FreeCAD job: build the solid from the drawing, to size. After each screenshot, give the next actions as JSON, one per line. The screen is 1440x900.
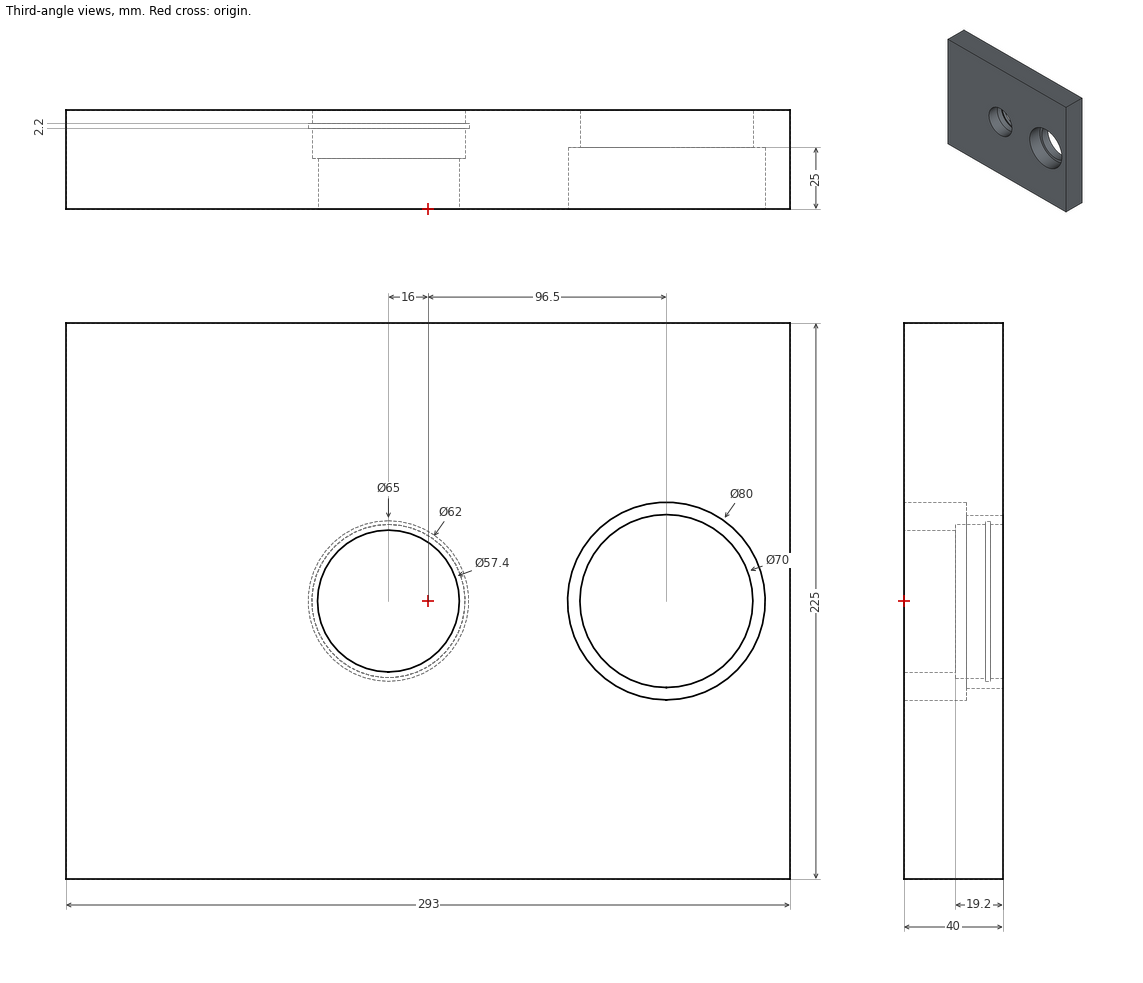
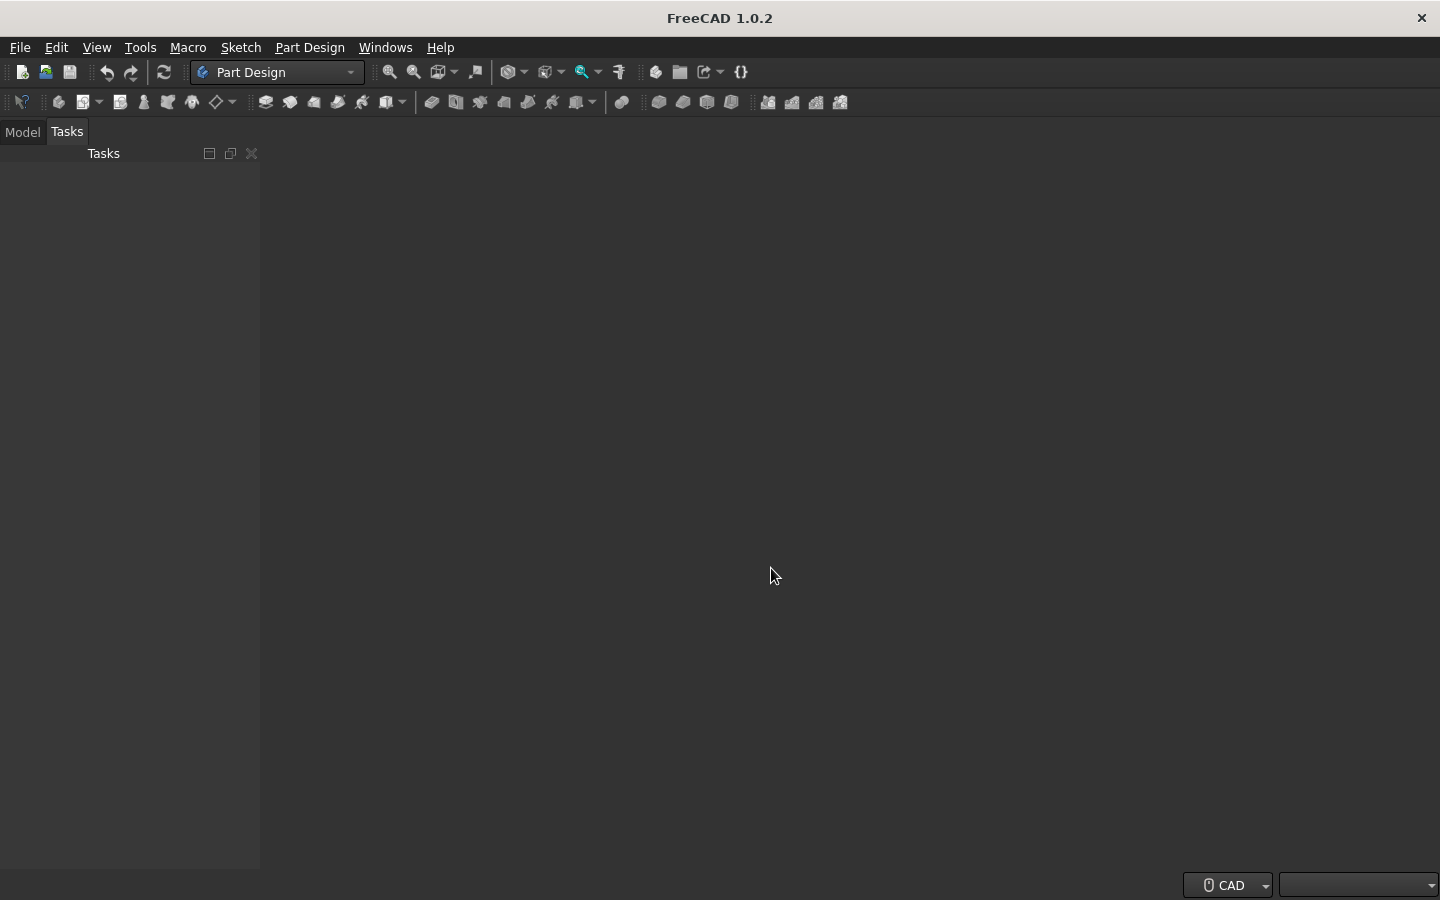
{"action": "left_click", "coordinate": [22, 72]}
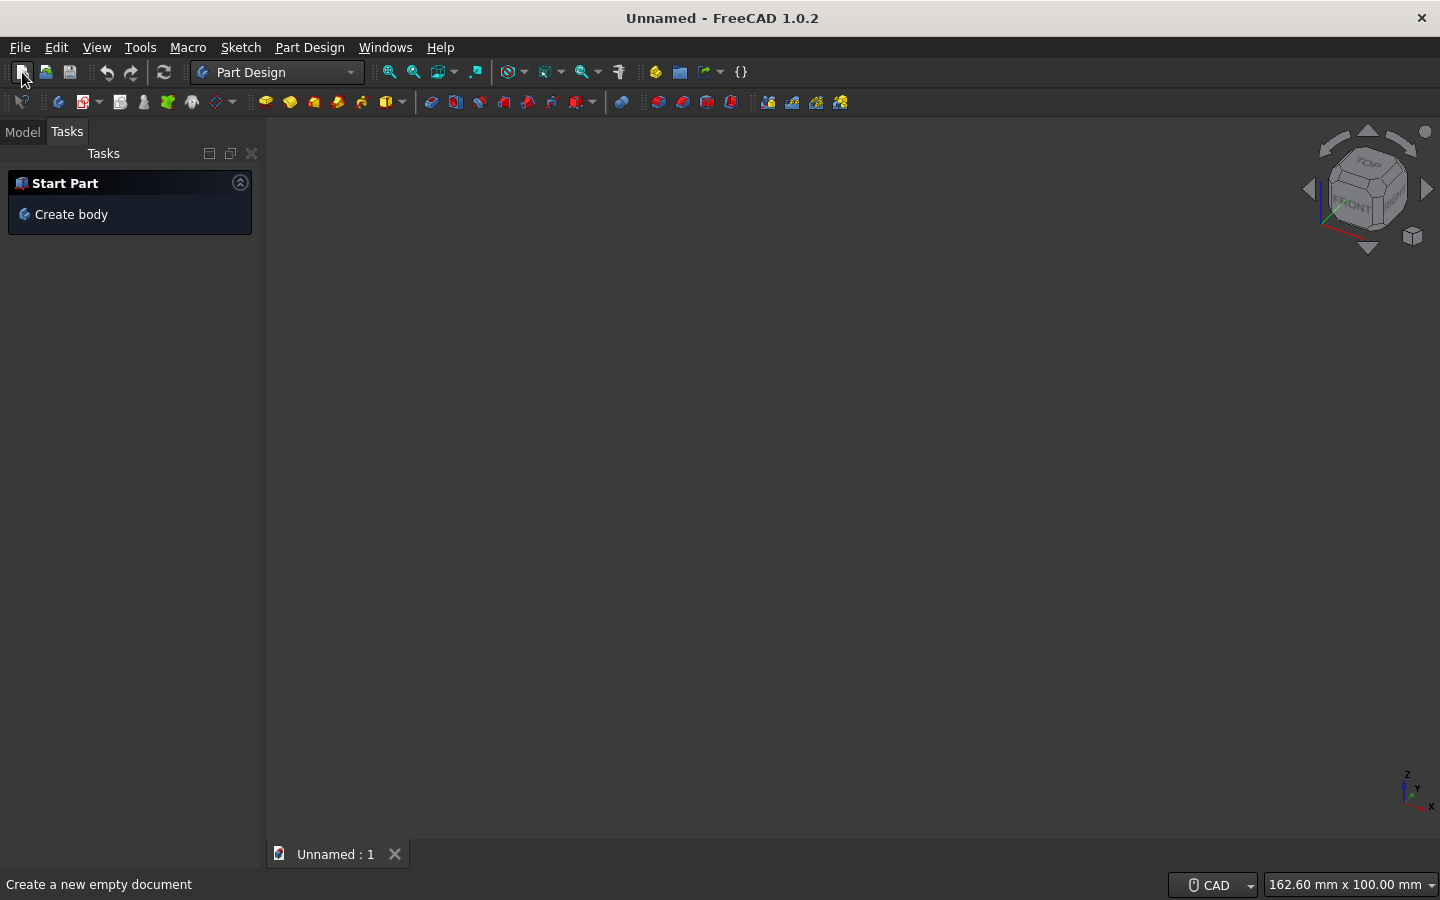
{"action": "left_click", "coordinate": [84, 102]}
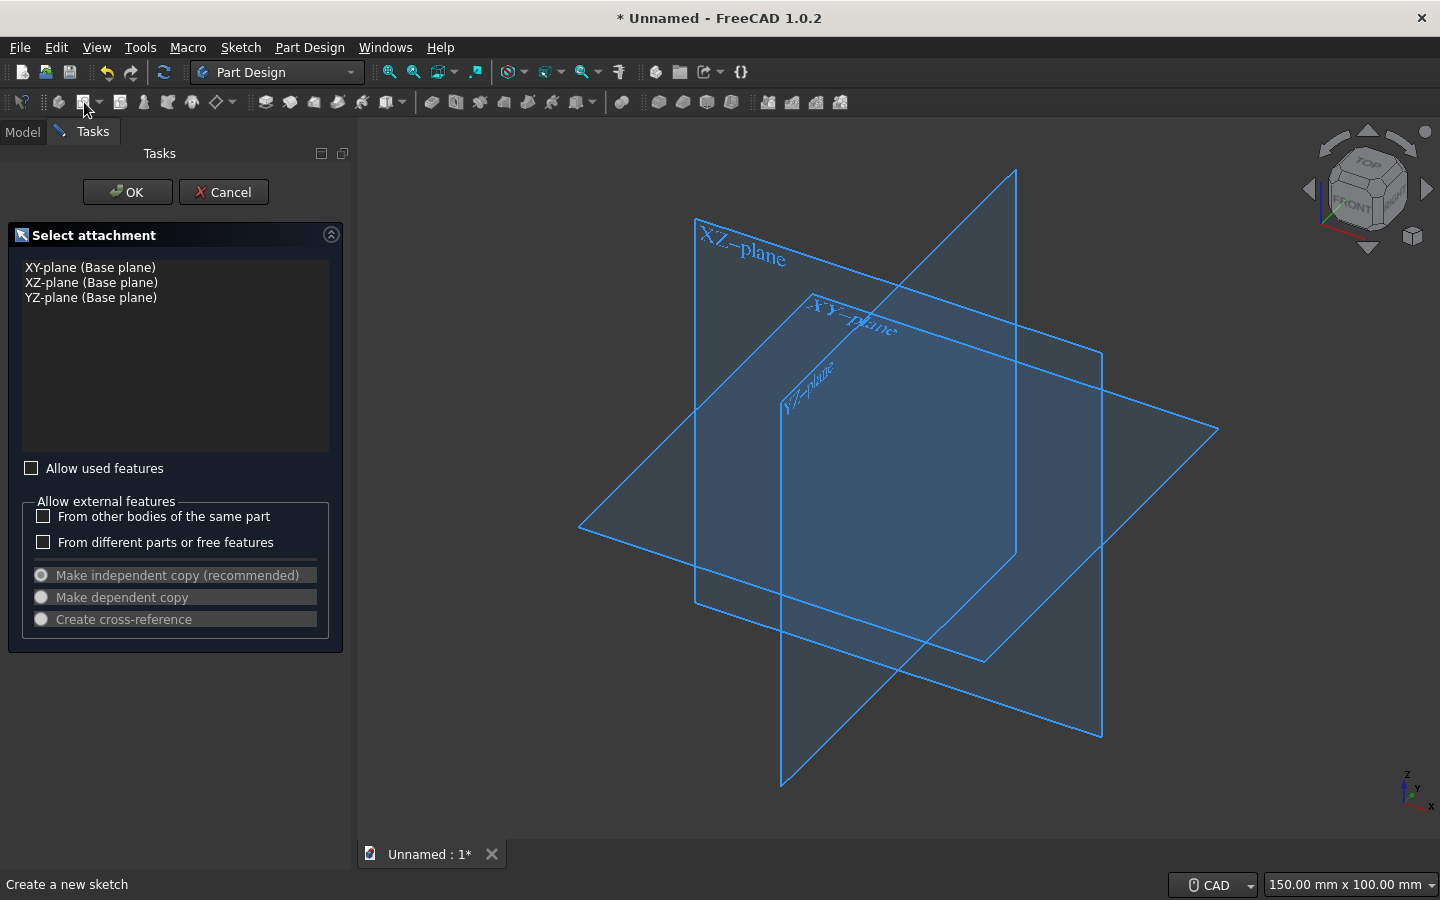
{"action": "left_click", "coordinate": [82, 282]}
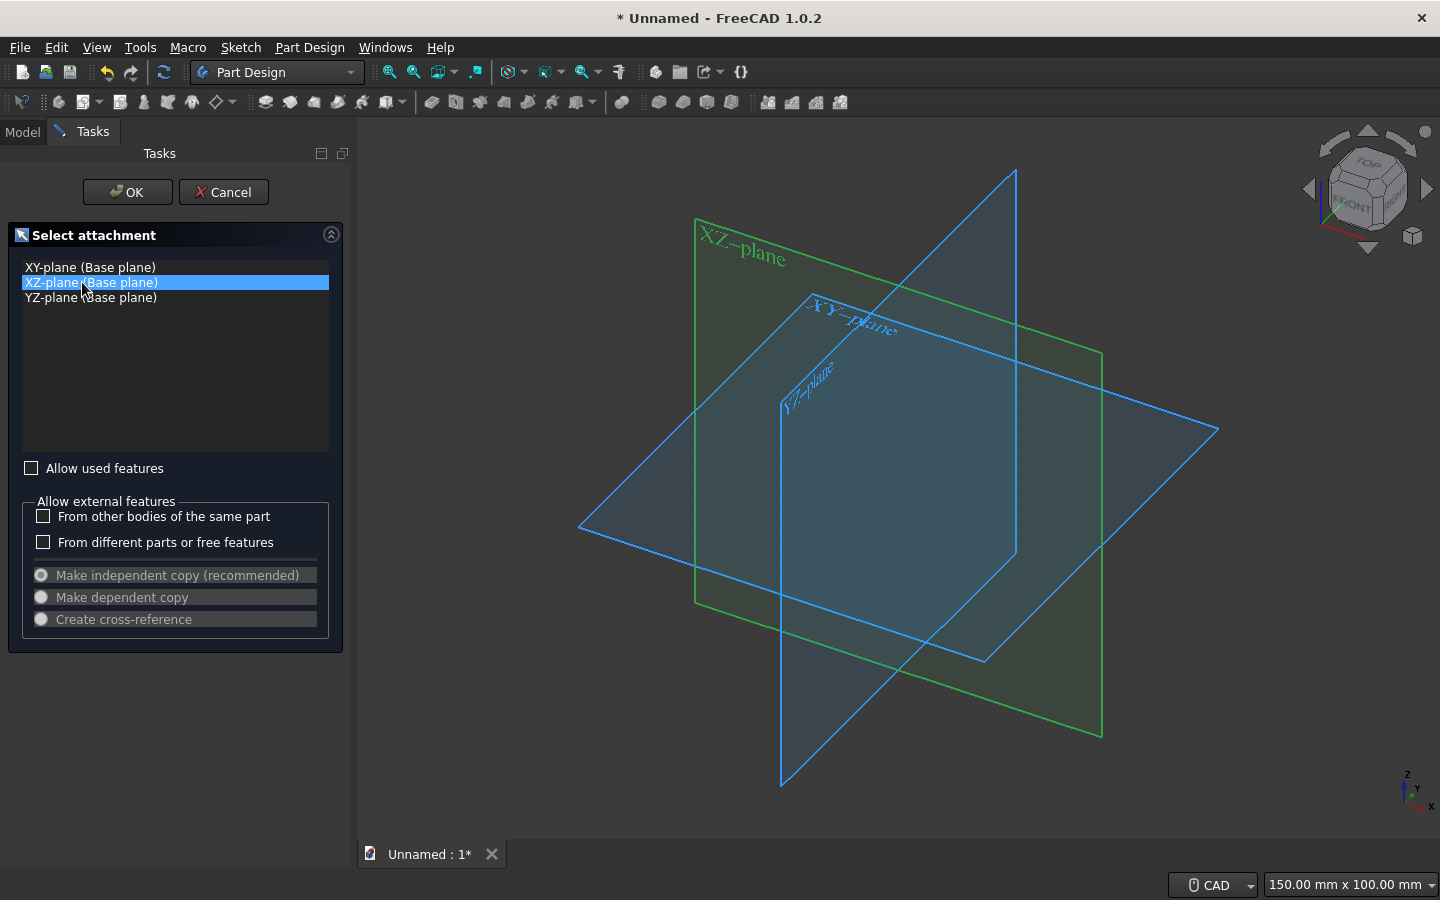
{"action": "left_click", "coordinate": [128, 192]}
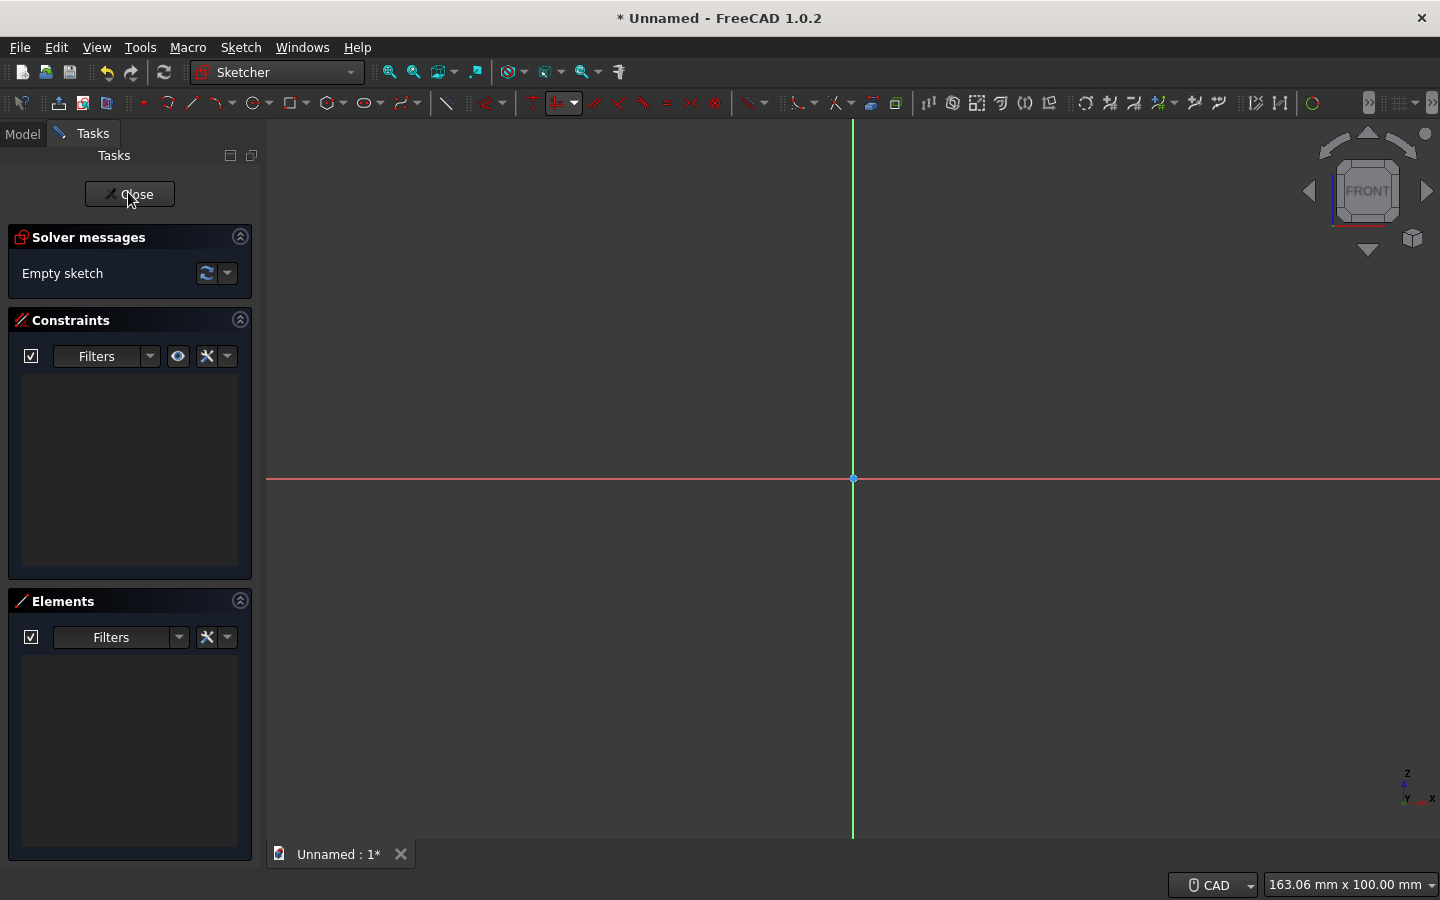
{"action": "scroll", "coordinate": [755, 479], "scroll_direction": "down", "scroll_amount": 6}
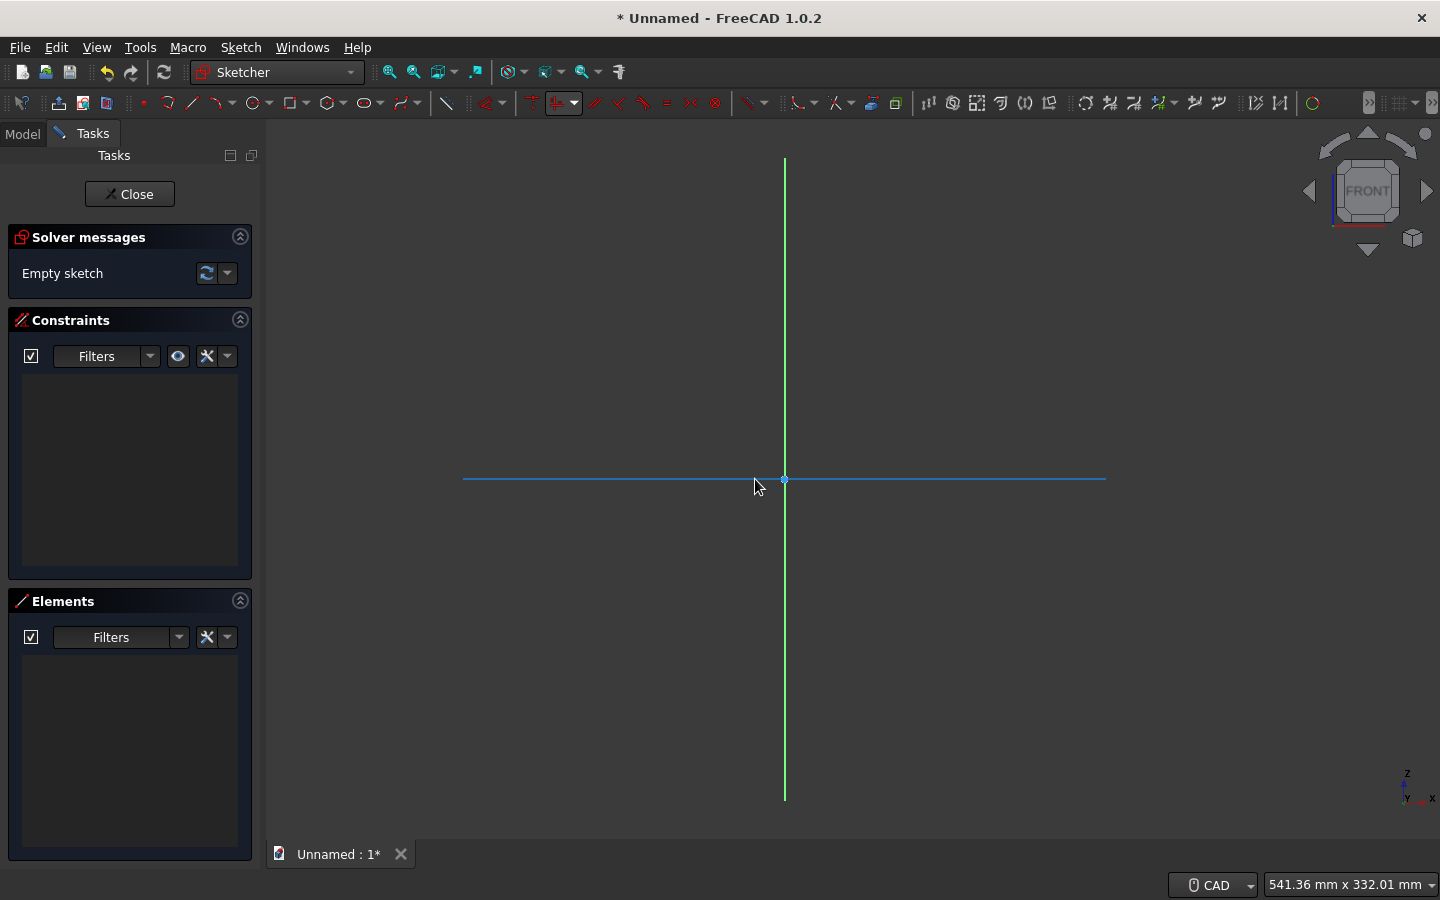
{"action": "left_click", "coordinate": [308, 104]}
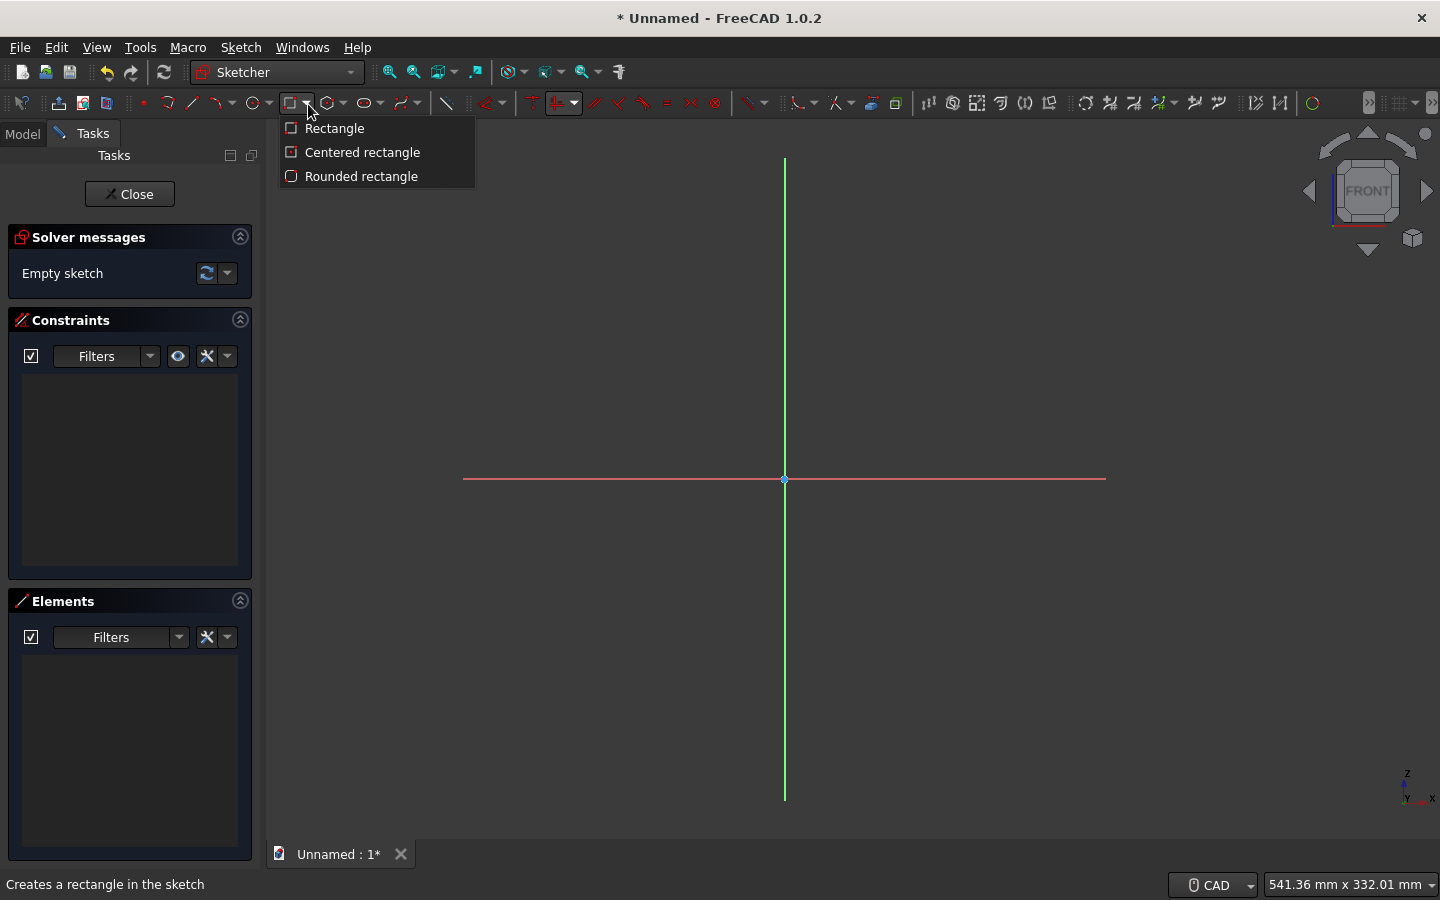
{"action": "left_click", "coordinate": [378, 152]}